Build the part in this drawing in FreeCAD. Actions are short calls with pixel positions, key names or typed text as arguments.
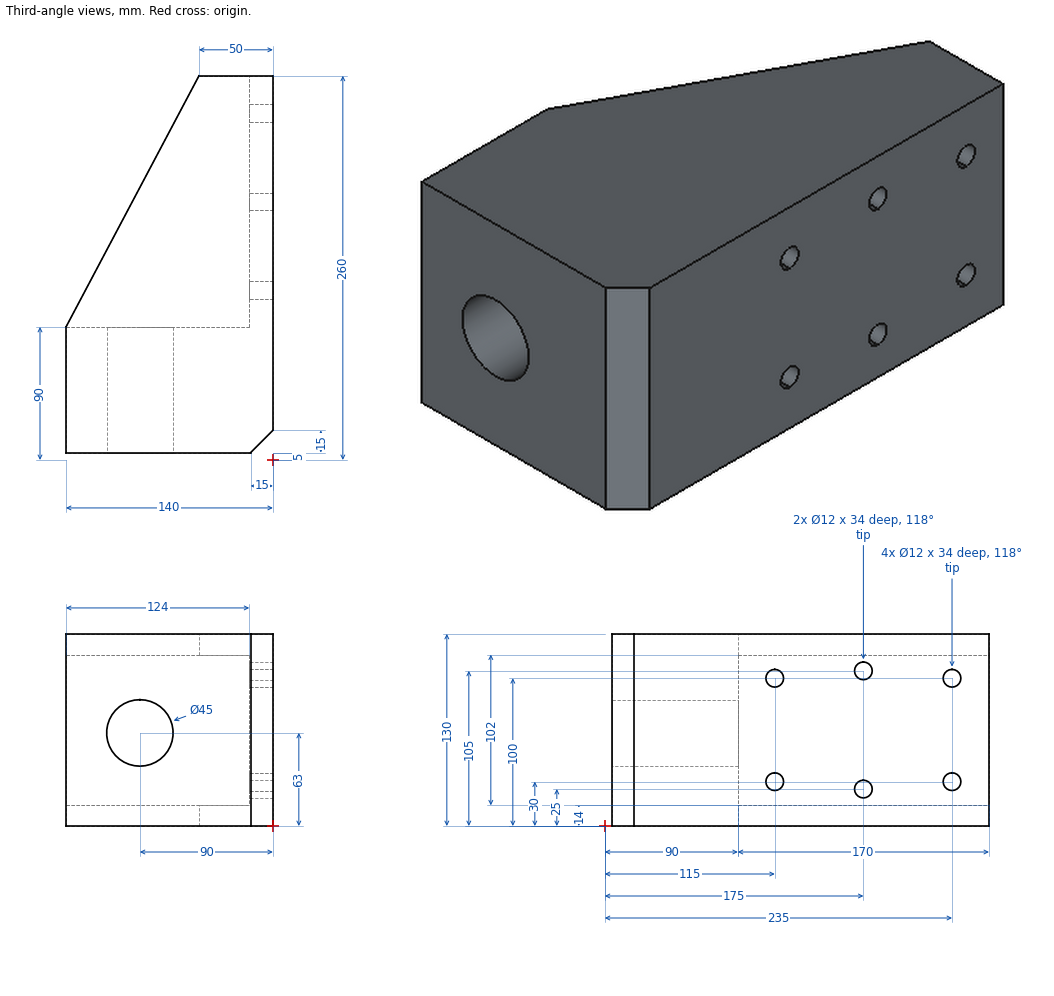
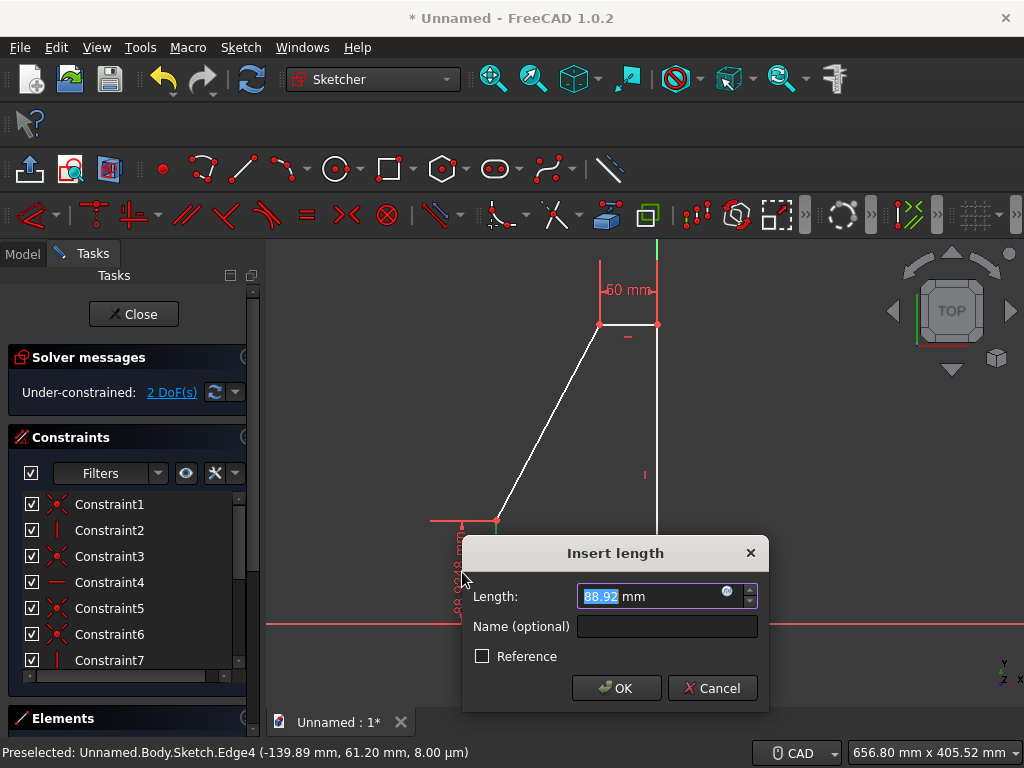
text(90)
key(Return)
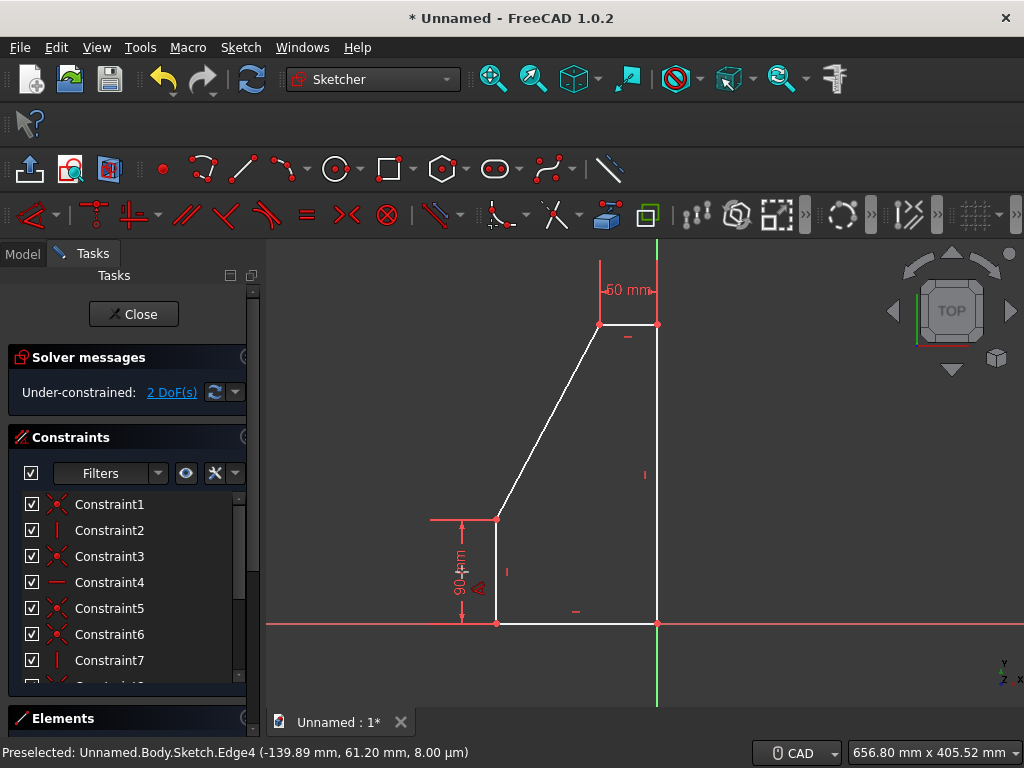
click(657, 534)
click(691, 474)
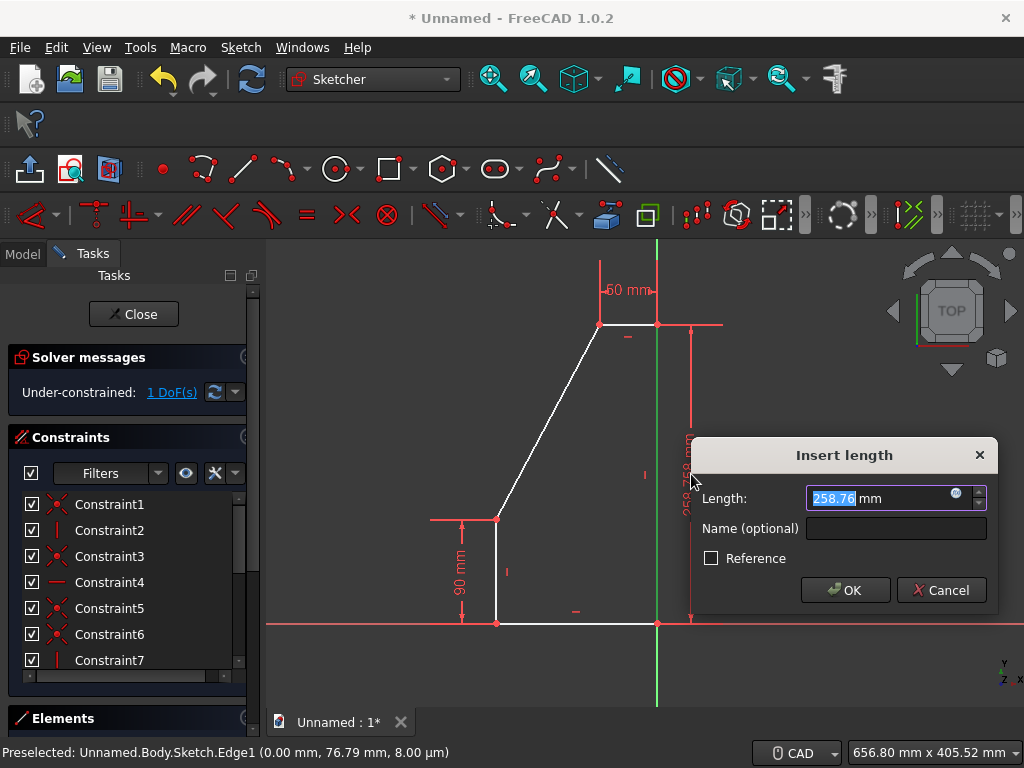
text(260)
key(Return)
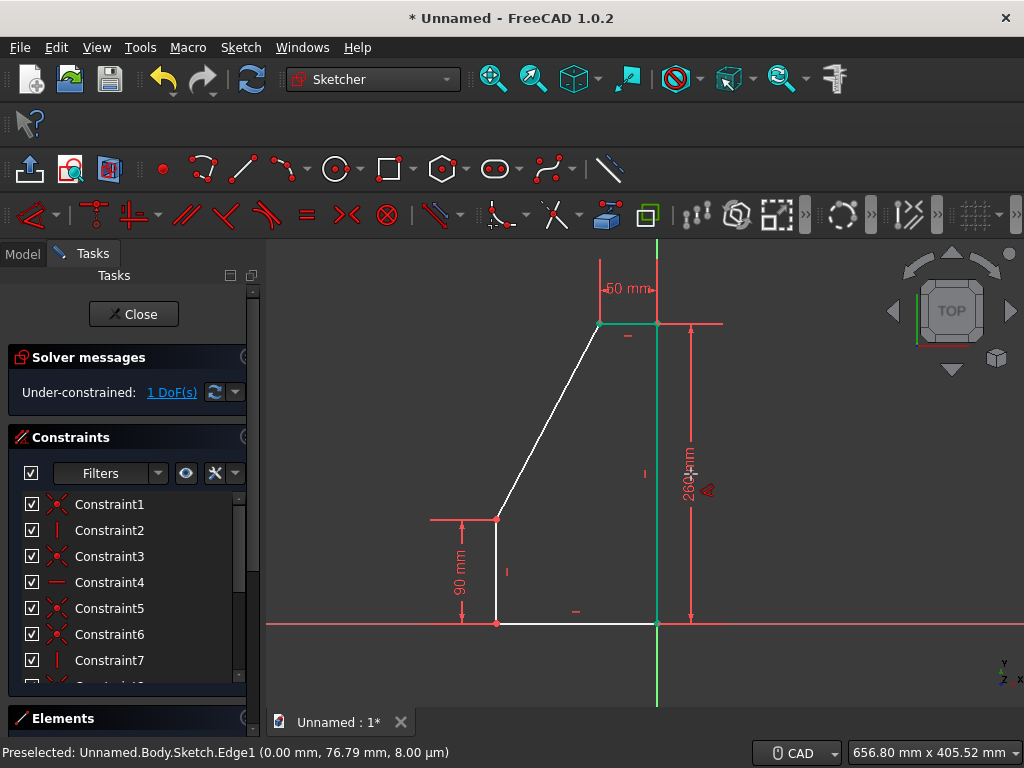
click(544, 624)
click(577, 658)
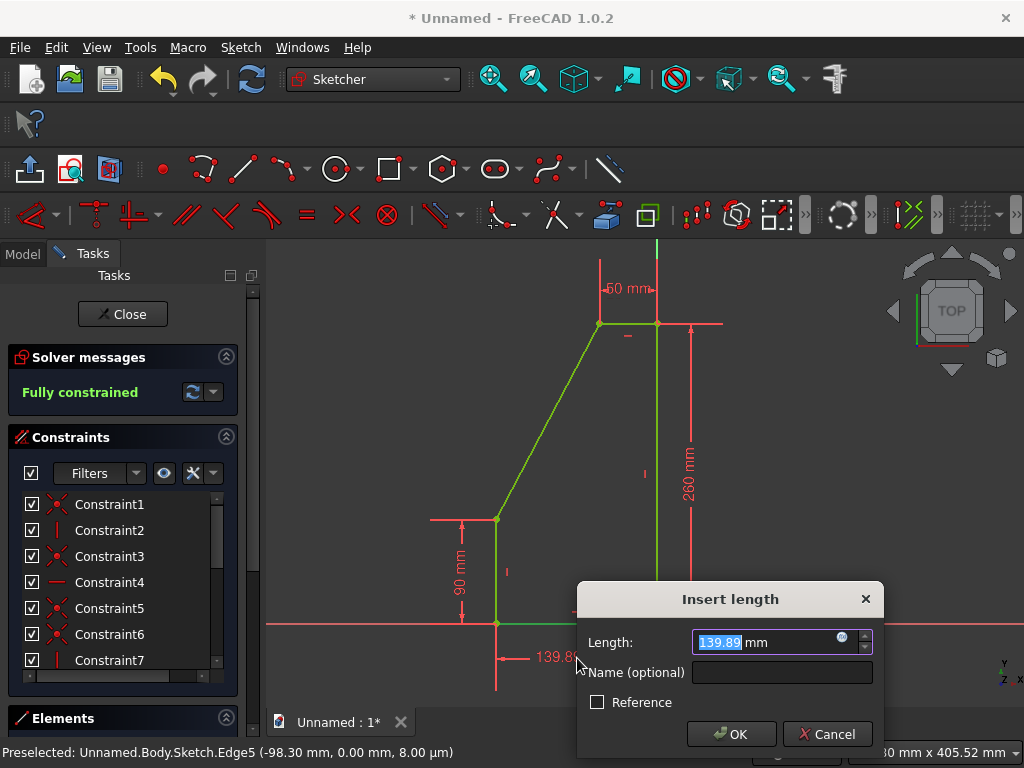
text(140)
key(Return)
key(Escape)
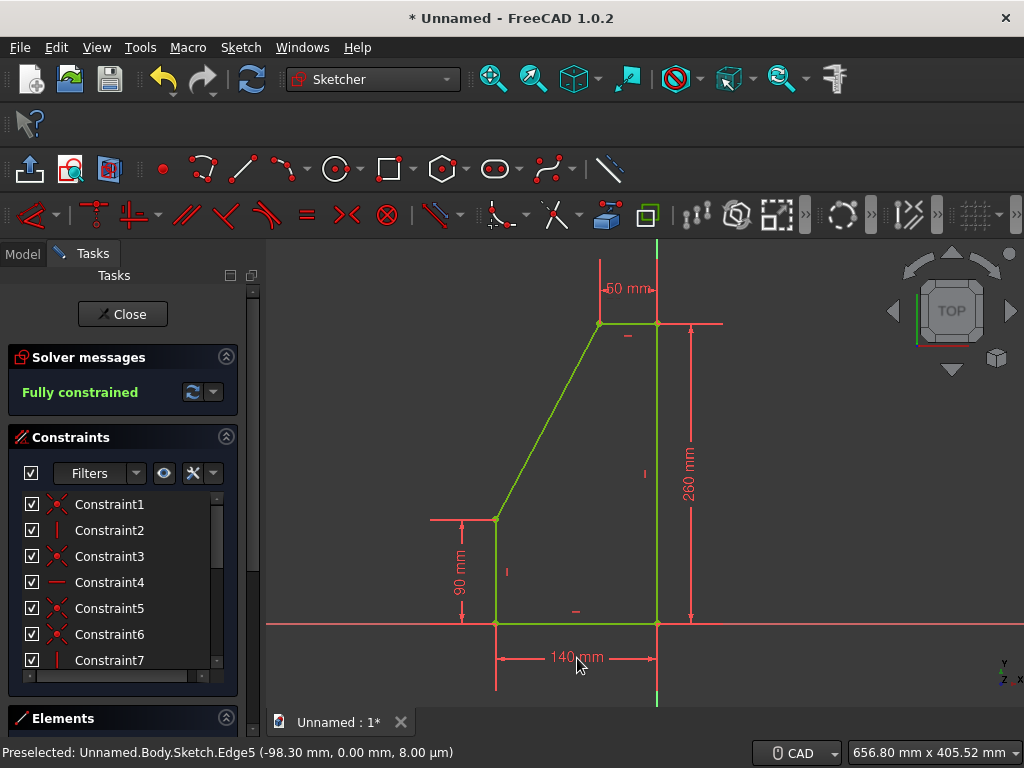
click(123, 314)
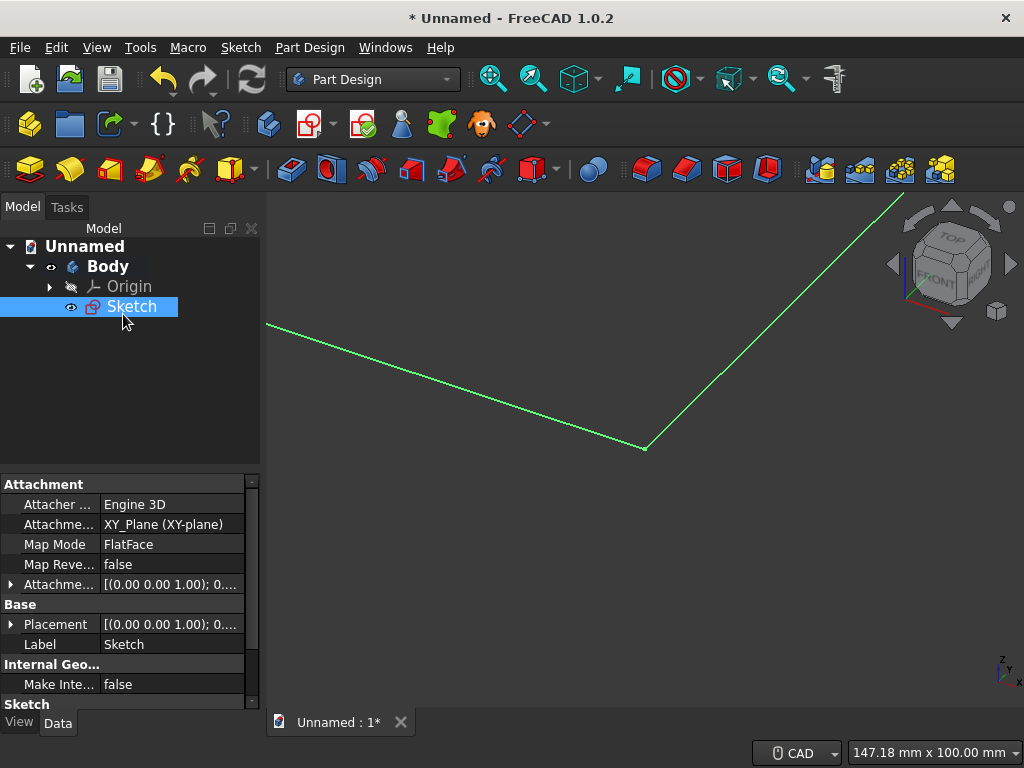
click(30, 170)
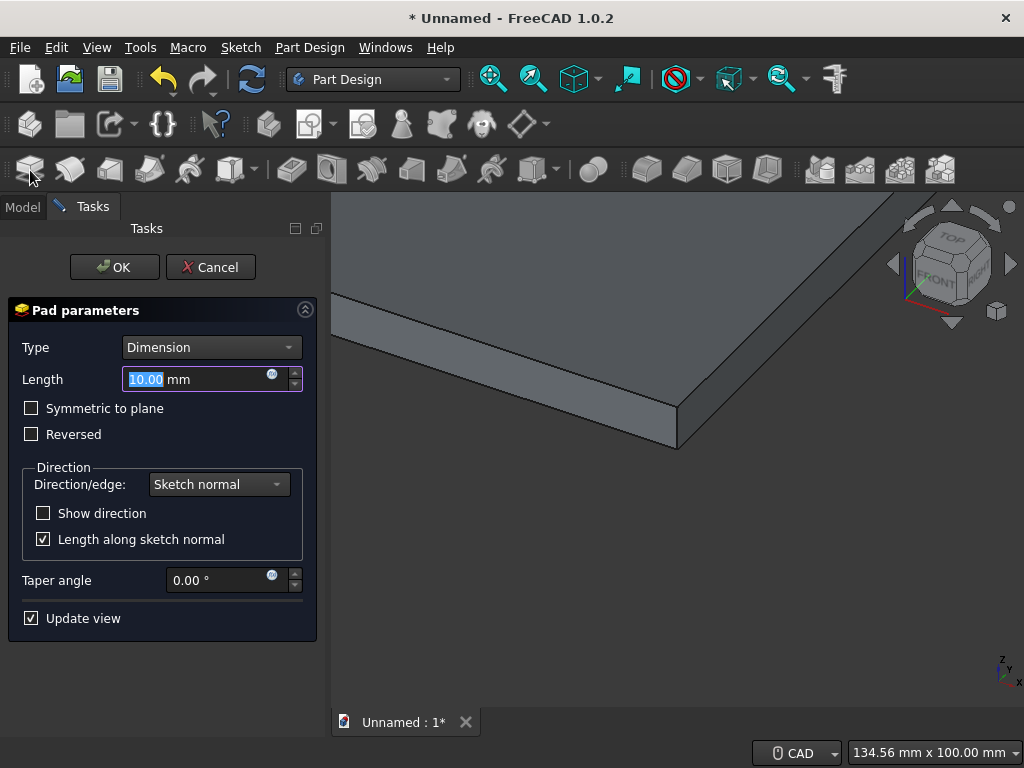
text(130)
key(Tab)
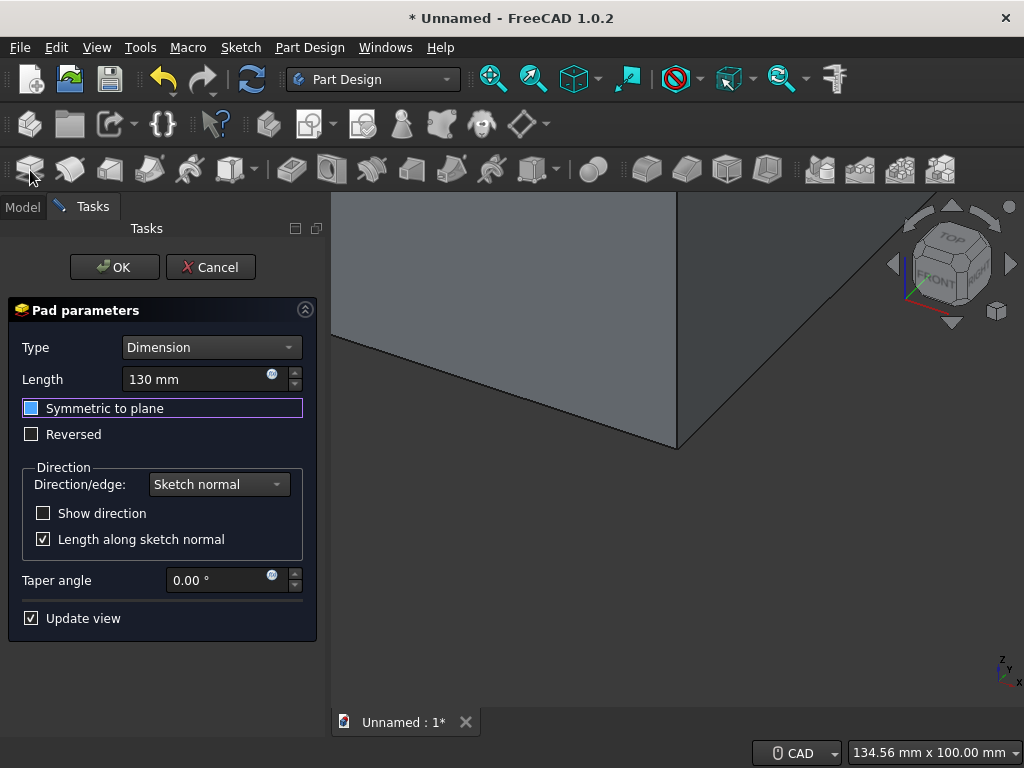
click(115, 267)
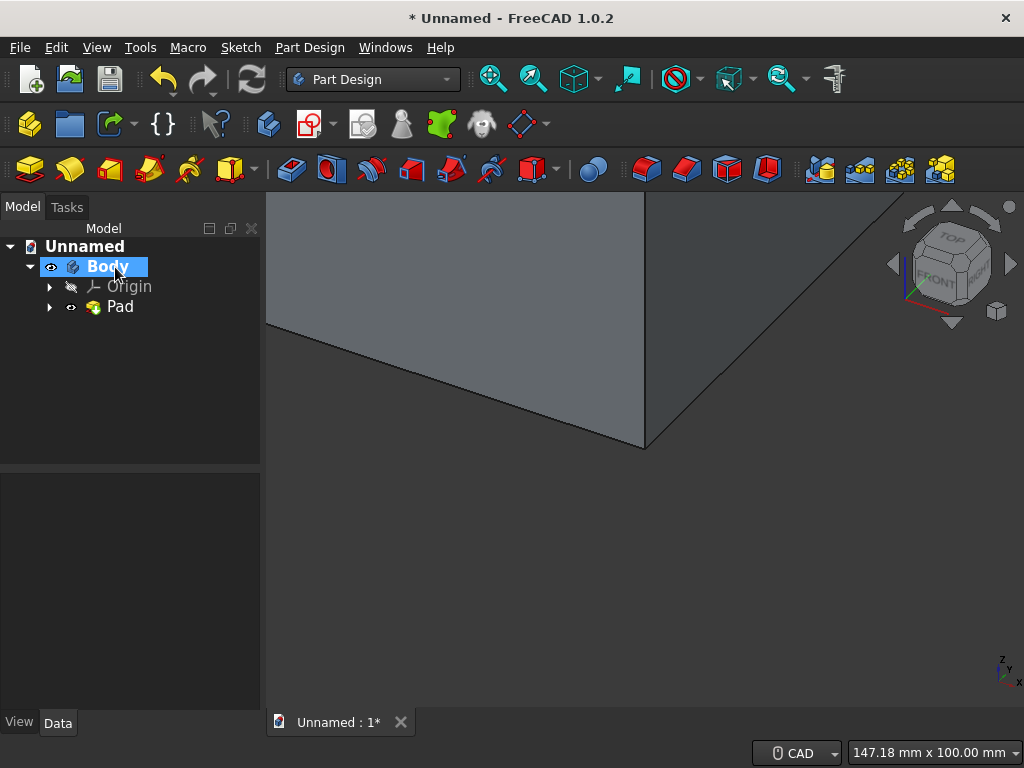
click(494, 80)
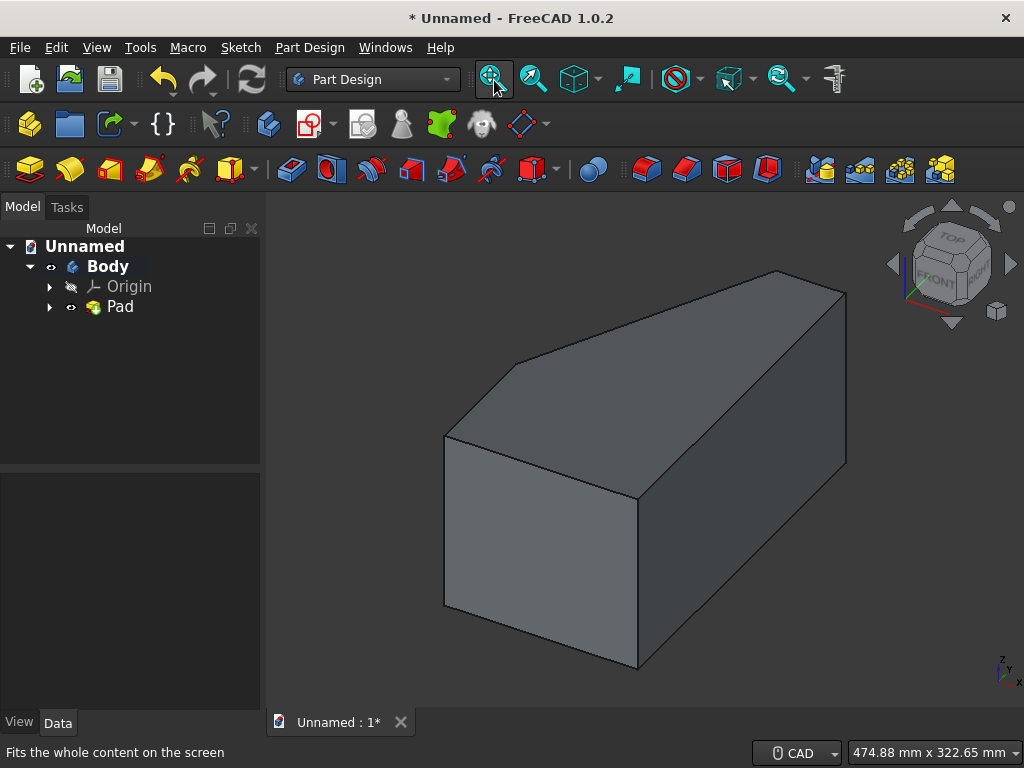
click(615, 393)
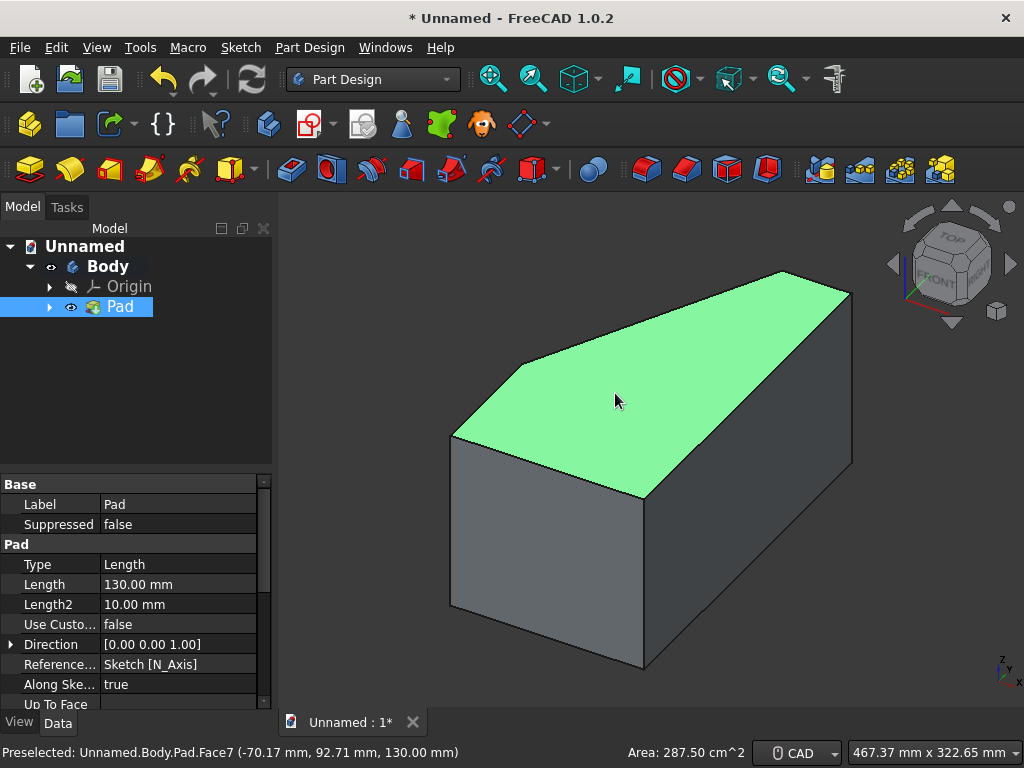
click(310, 124)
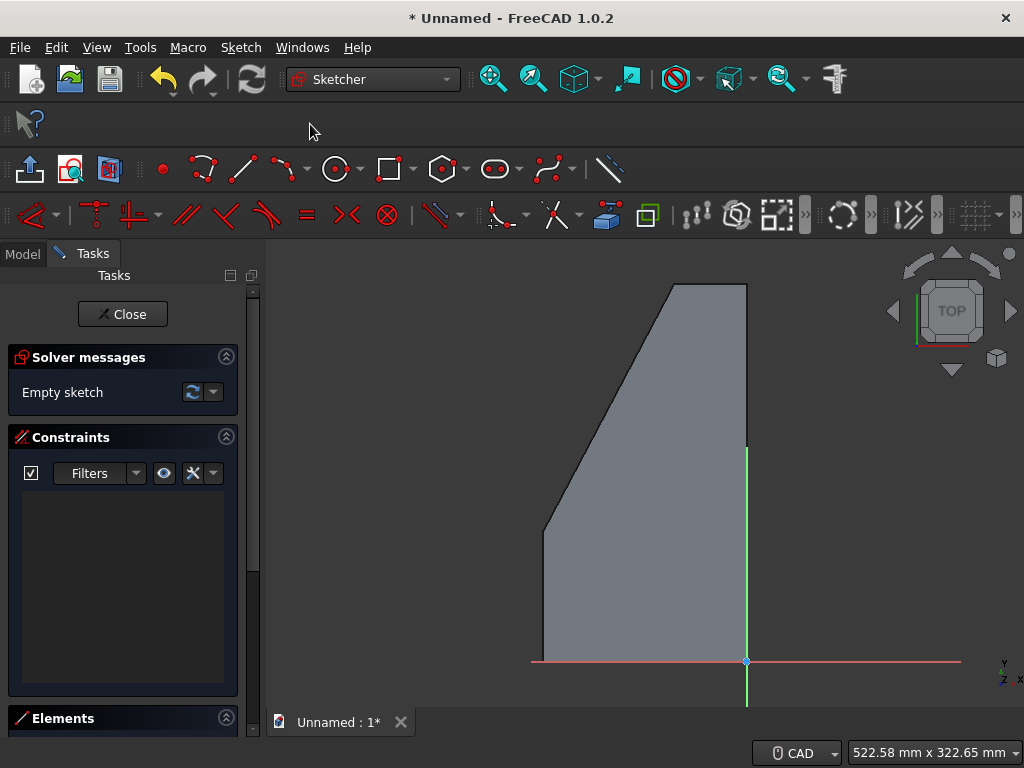
scroll(728, 679, up, 3)